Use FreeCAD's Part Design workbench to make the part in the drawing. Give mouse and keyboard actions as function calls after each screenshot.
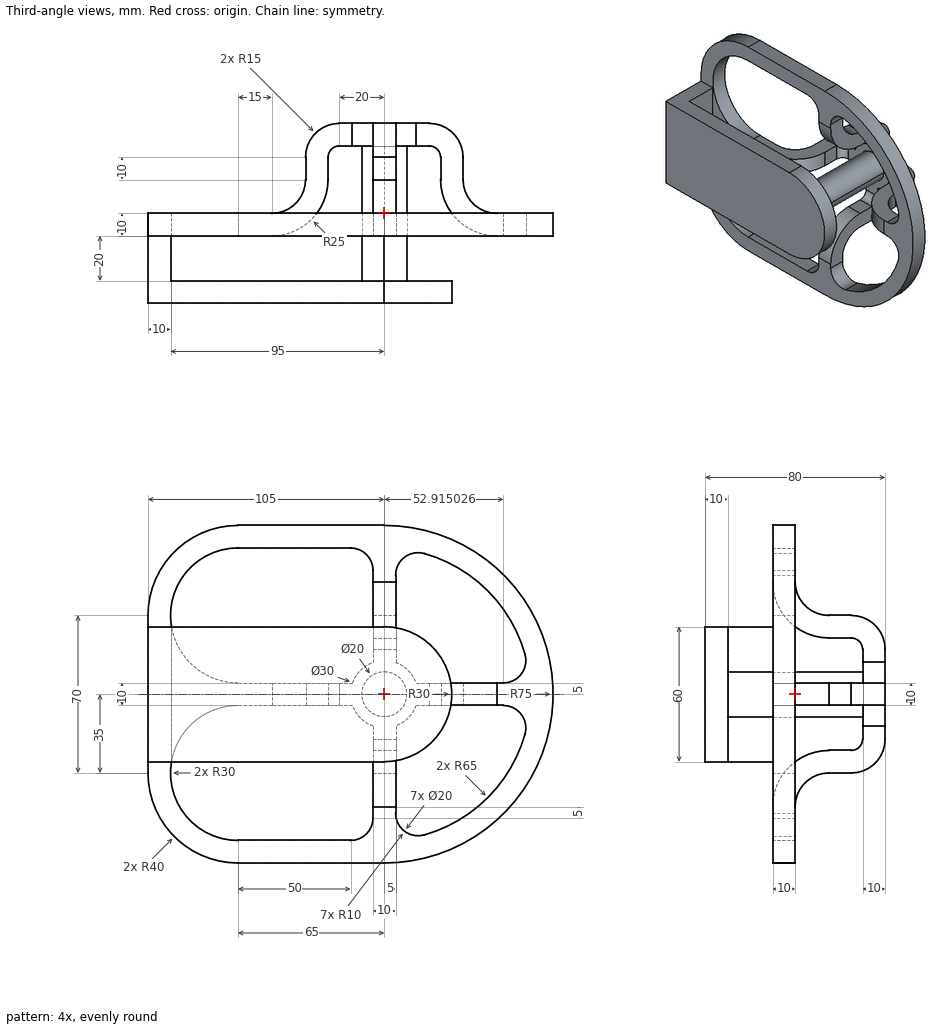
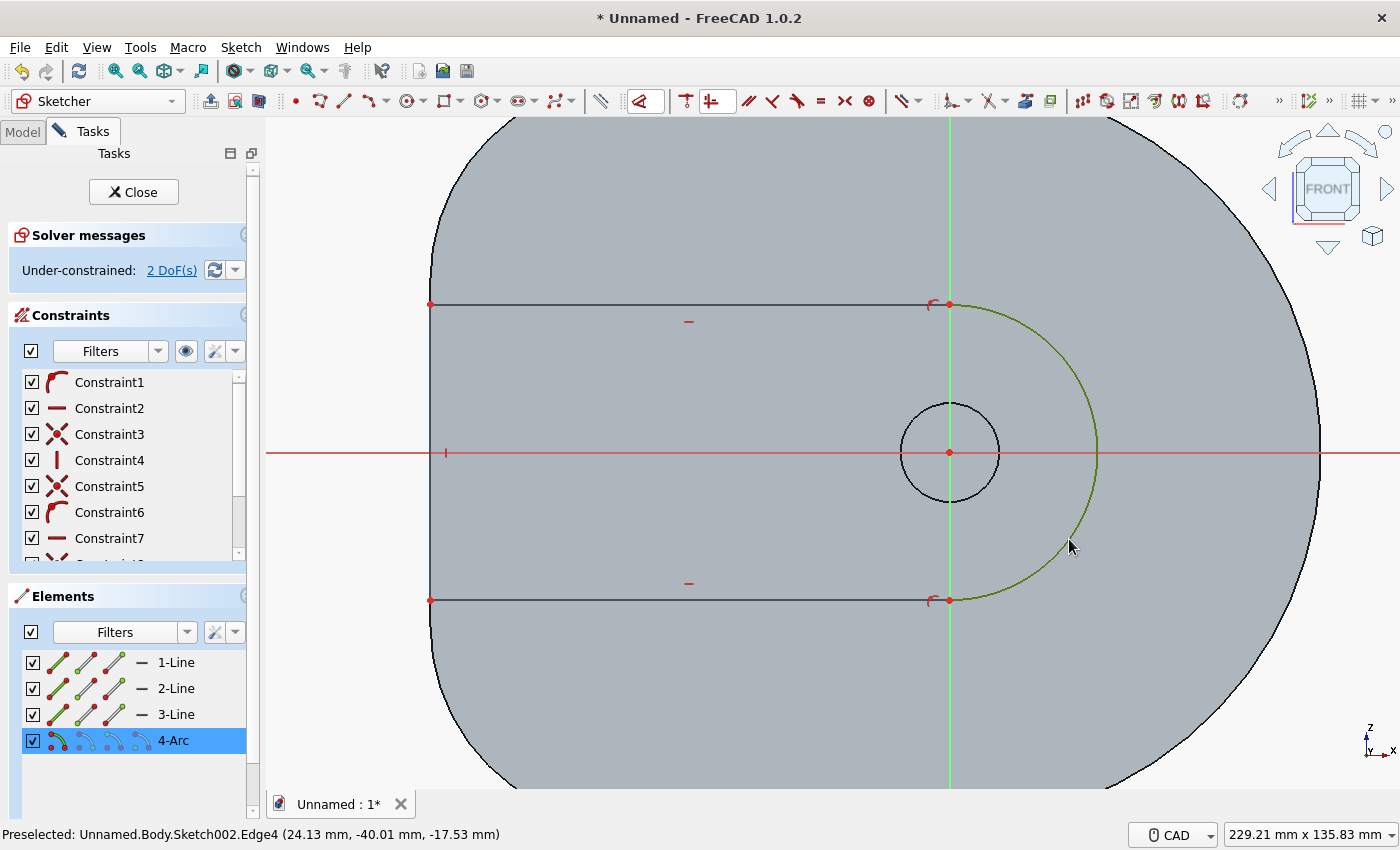
key(k)
key(r)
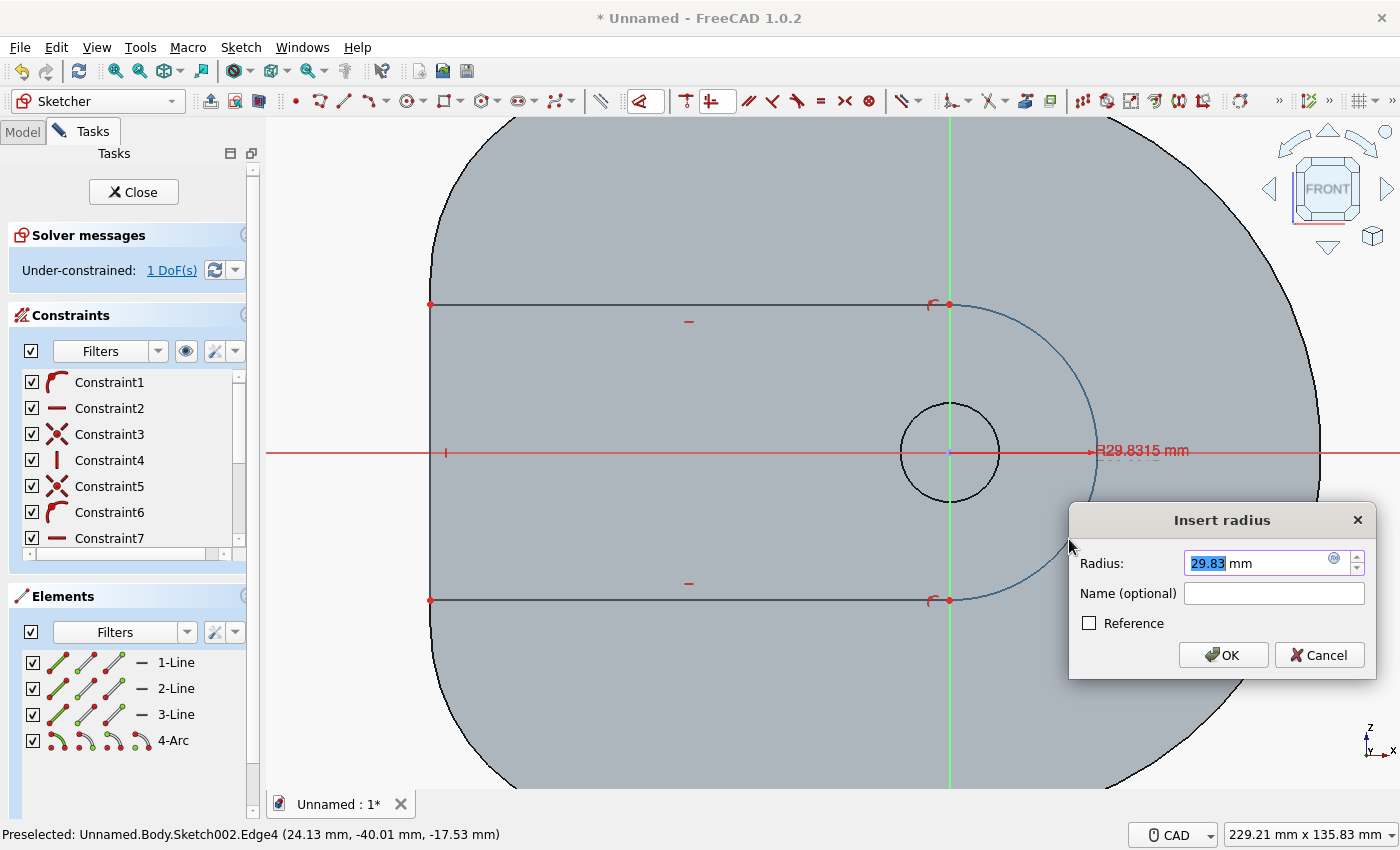
text(30)
key(Return)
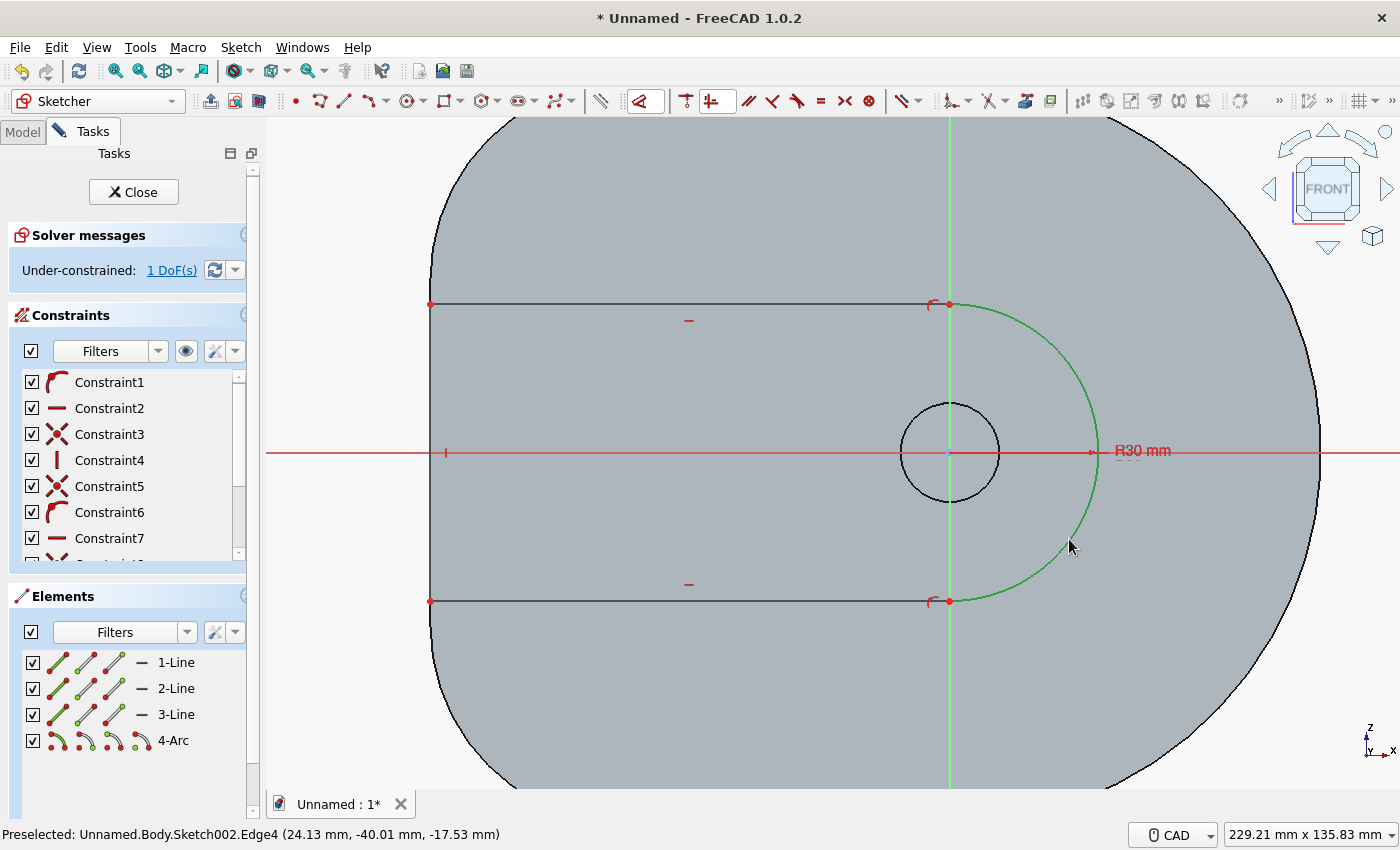
click(794, 304)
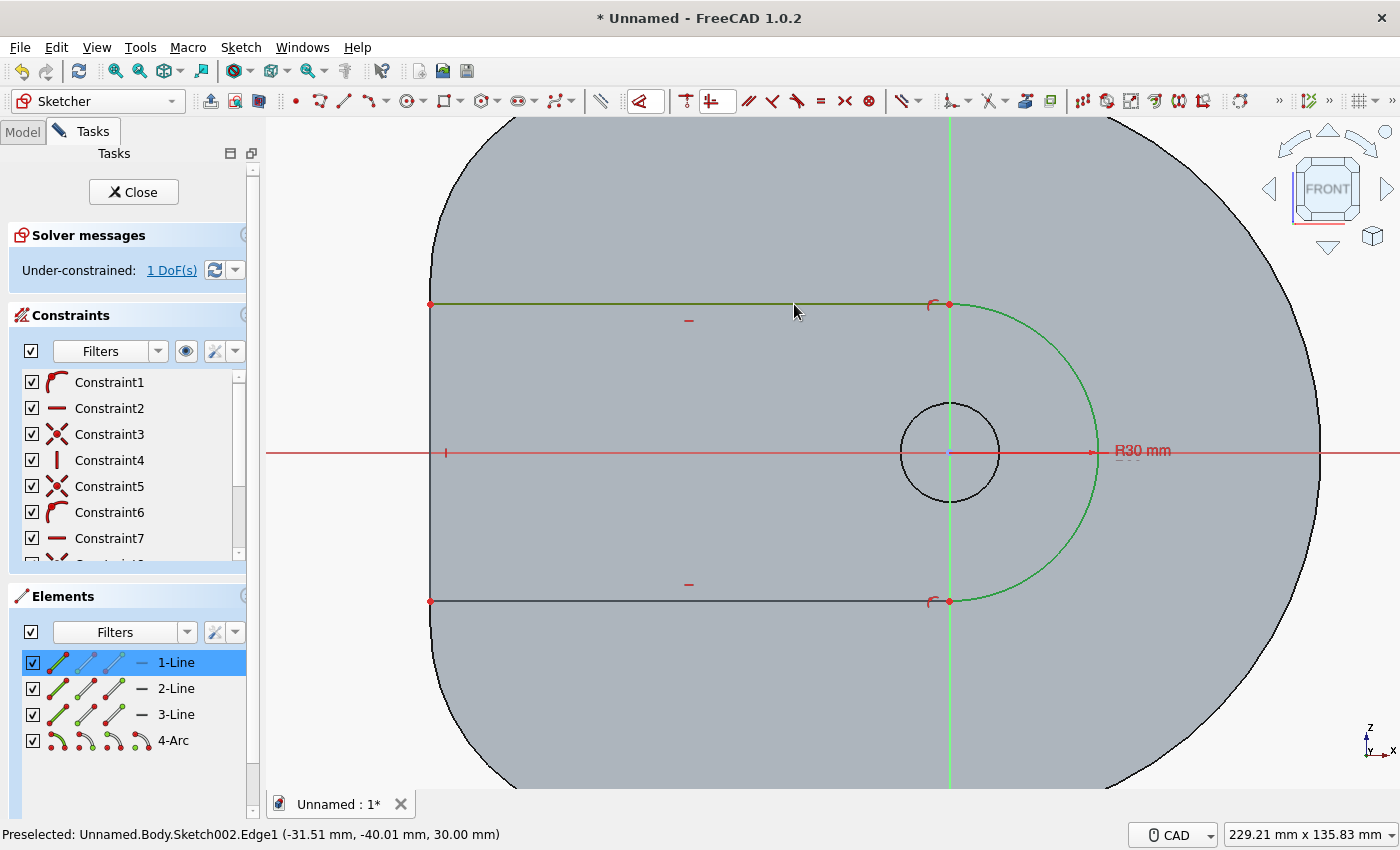
key(l)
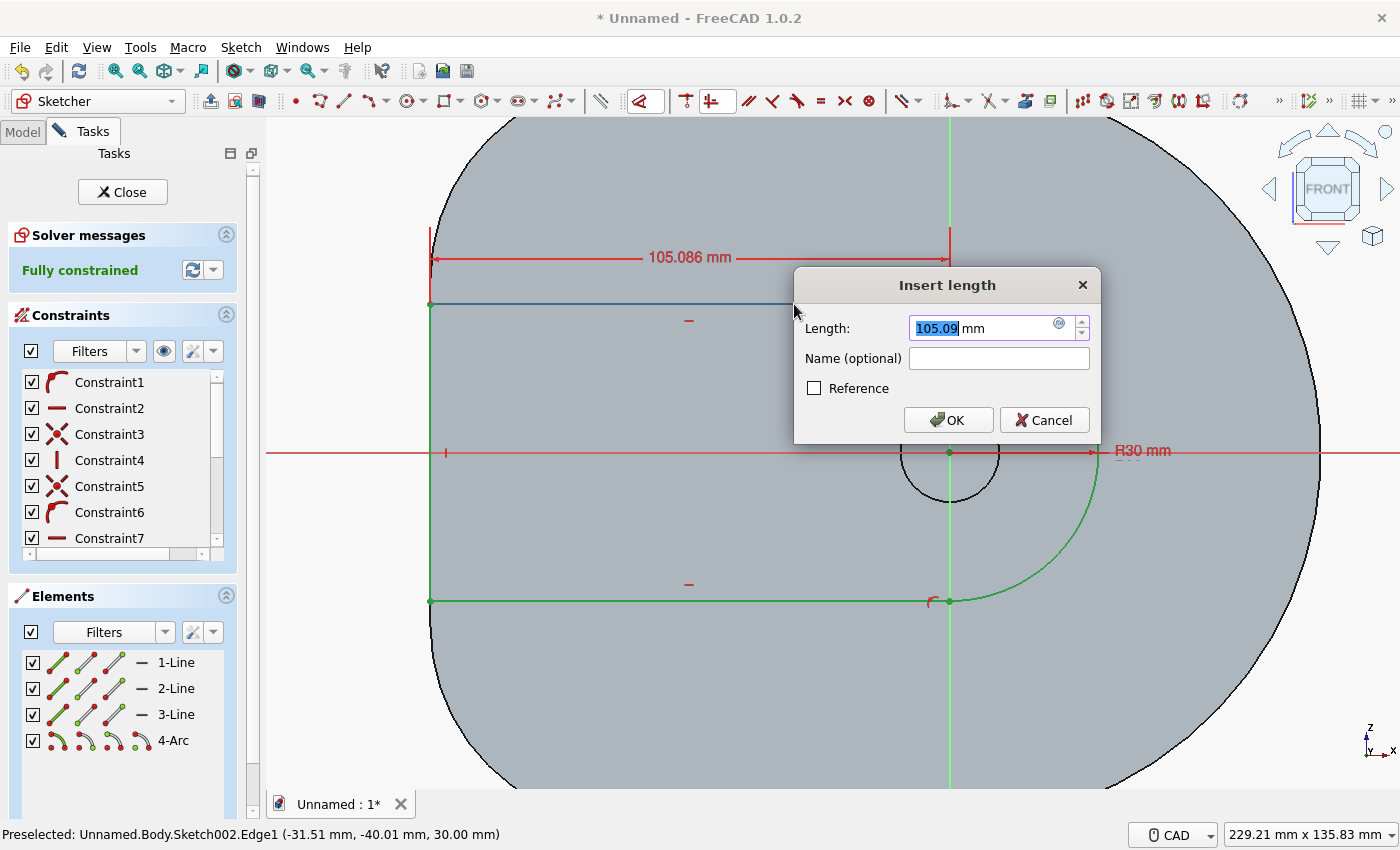
text(105)
key(Return)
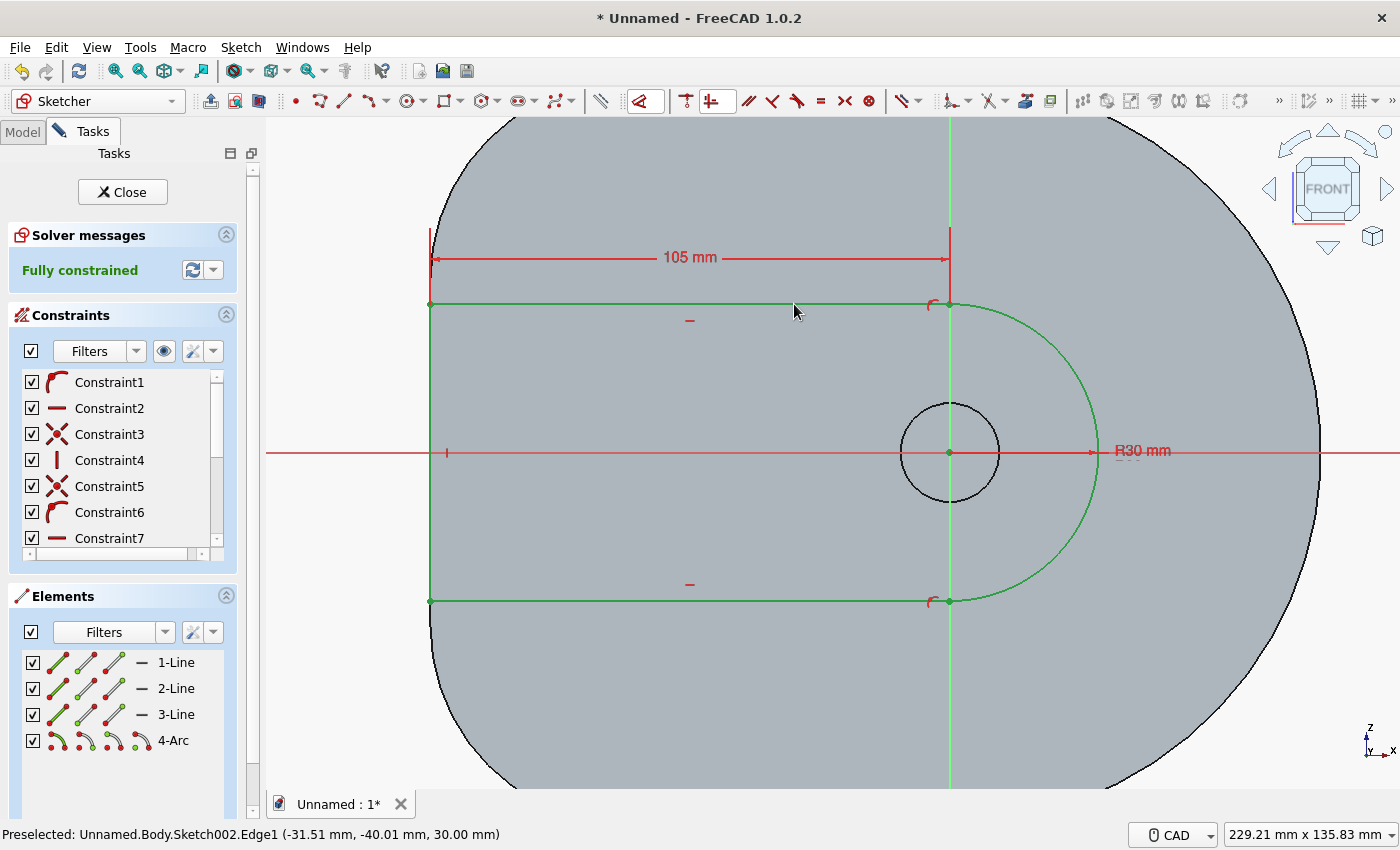
click(123, 192)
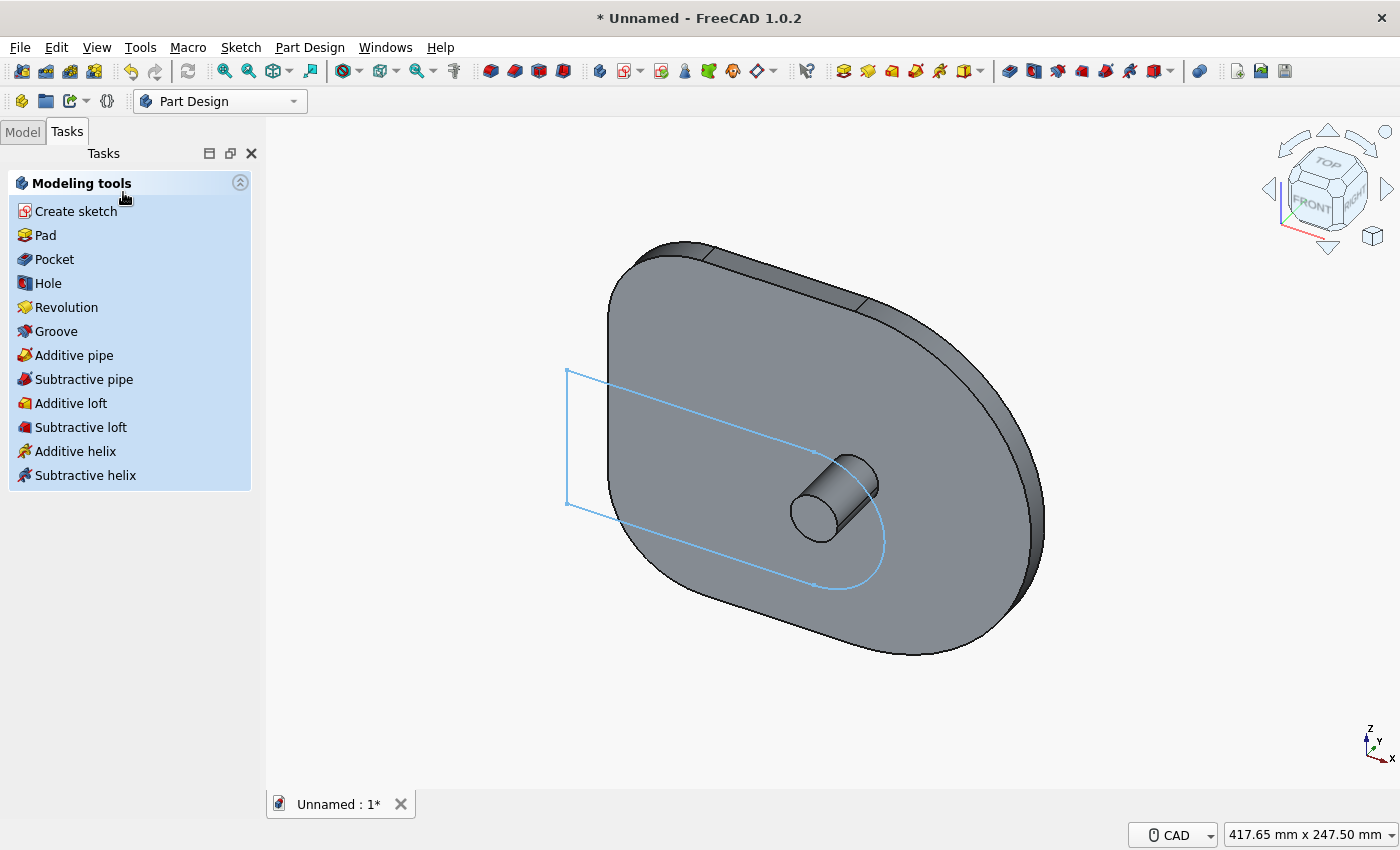
click(844, 72)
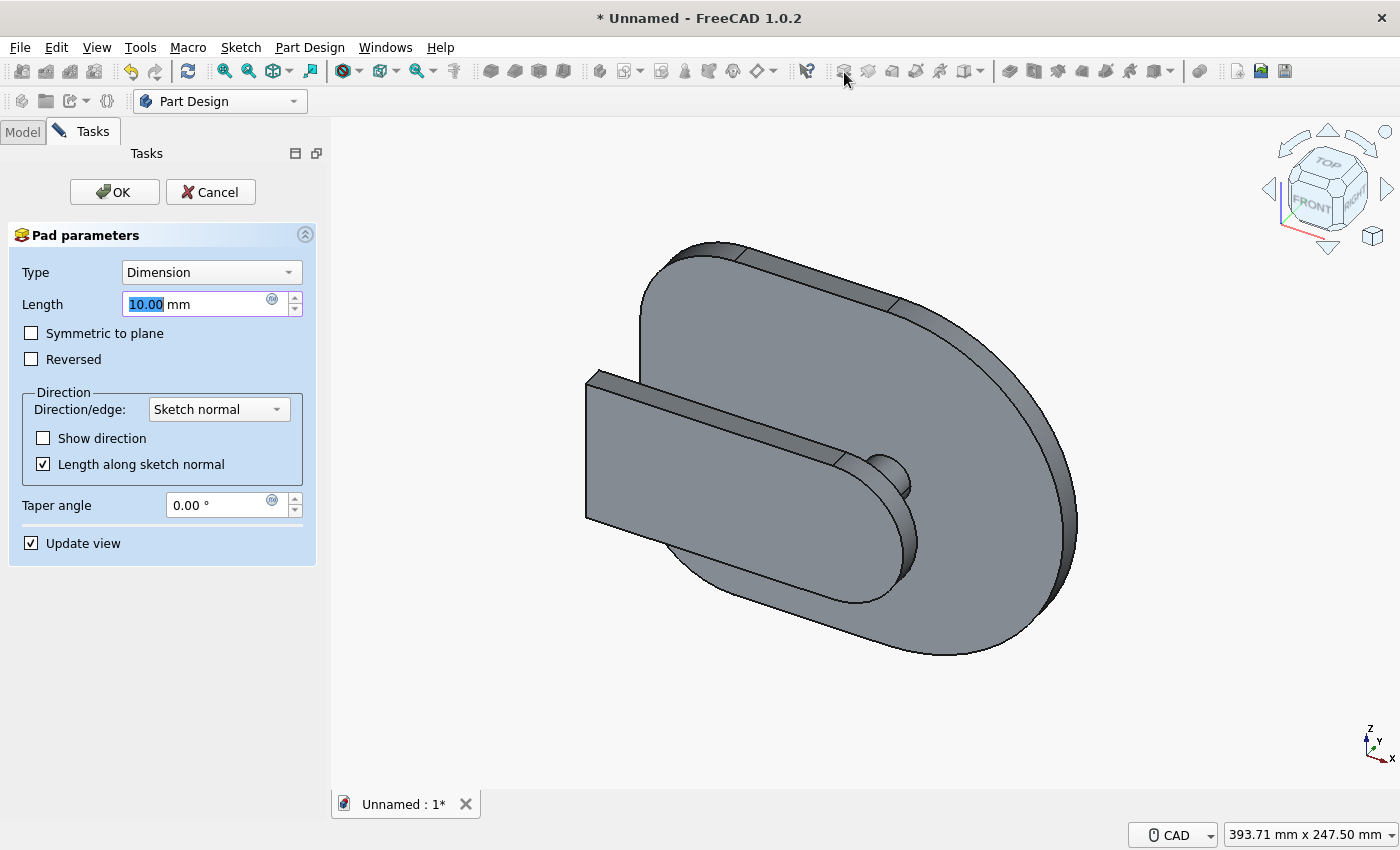
text(10)
key(Tab)